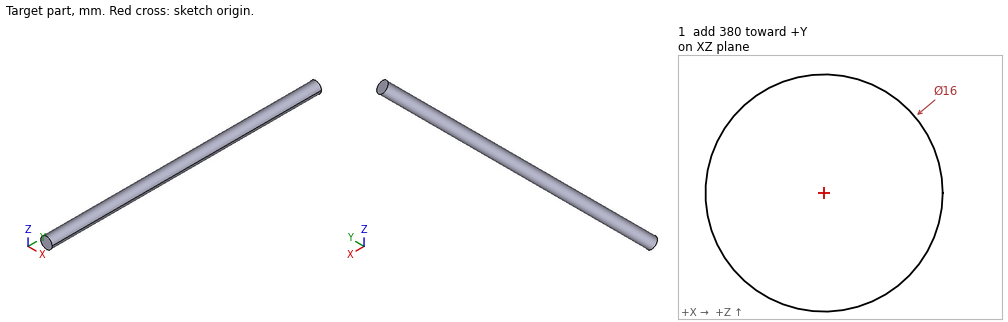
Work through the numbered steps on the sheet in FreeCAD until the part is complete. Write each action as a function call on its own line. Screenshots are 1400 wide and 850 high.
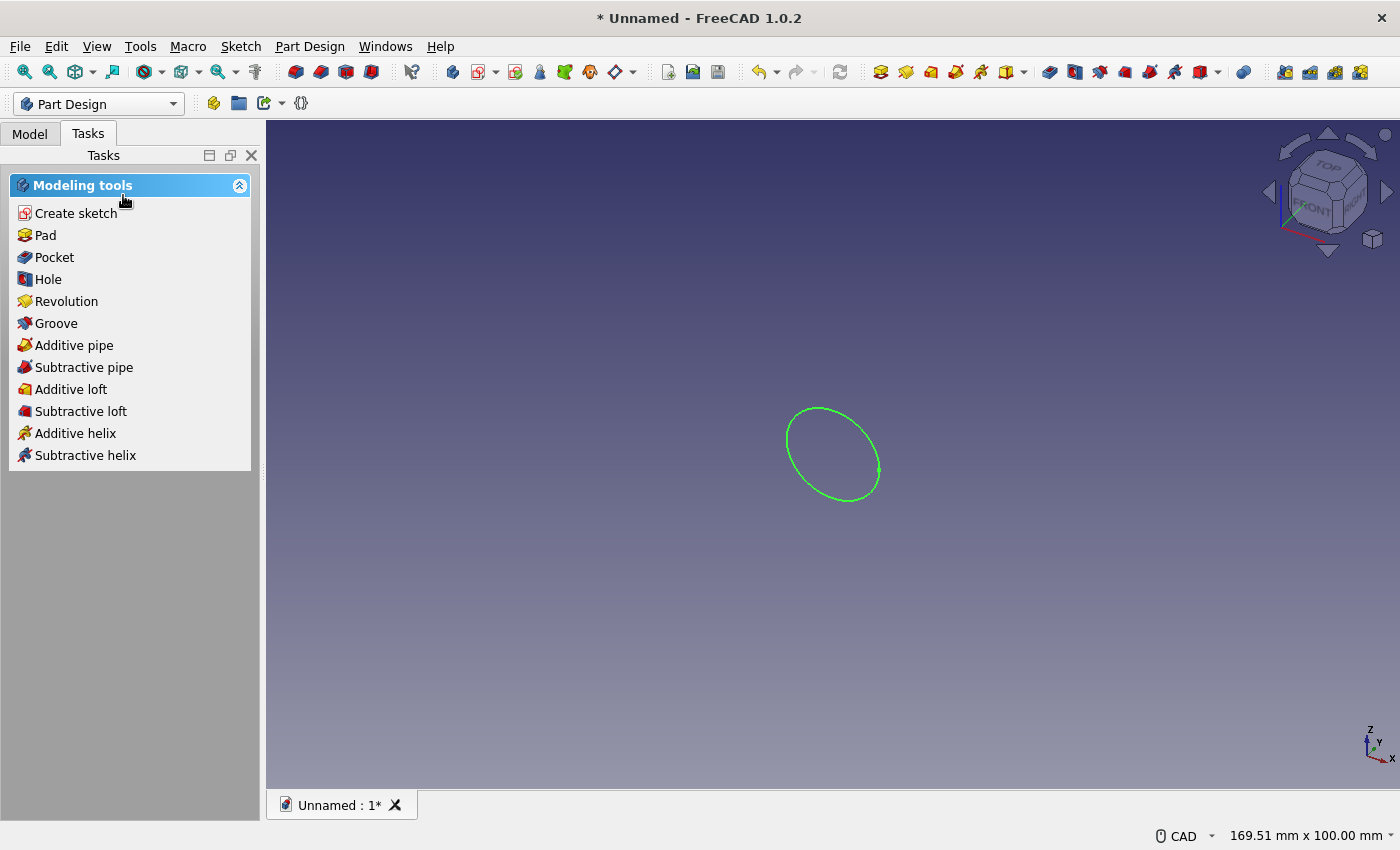
click(881, 72)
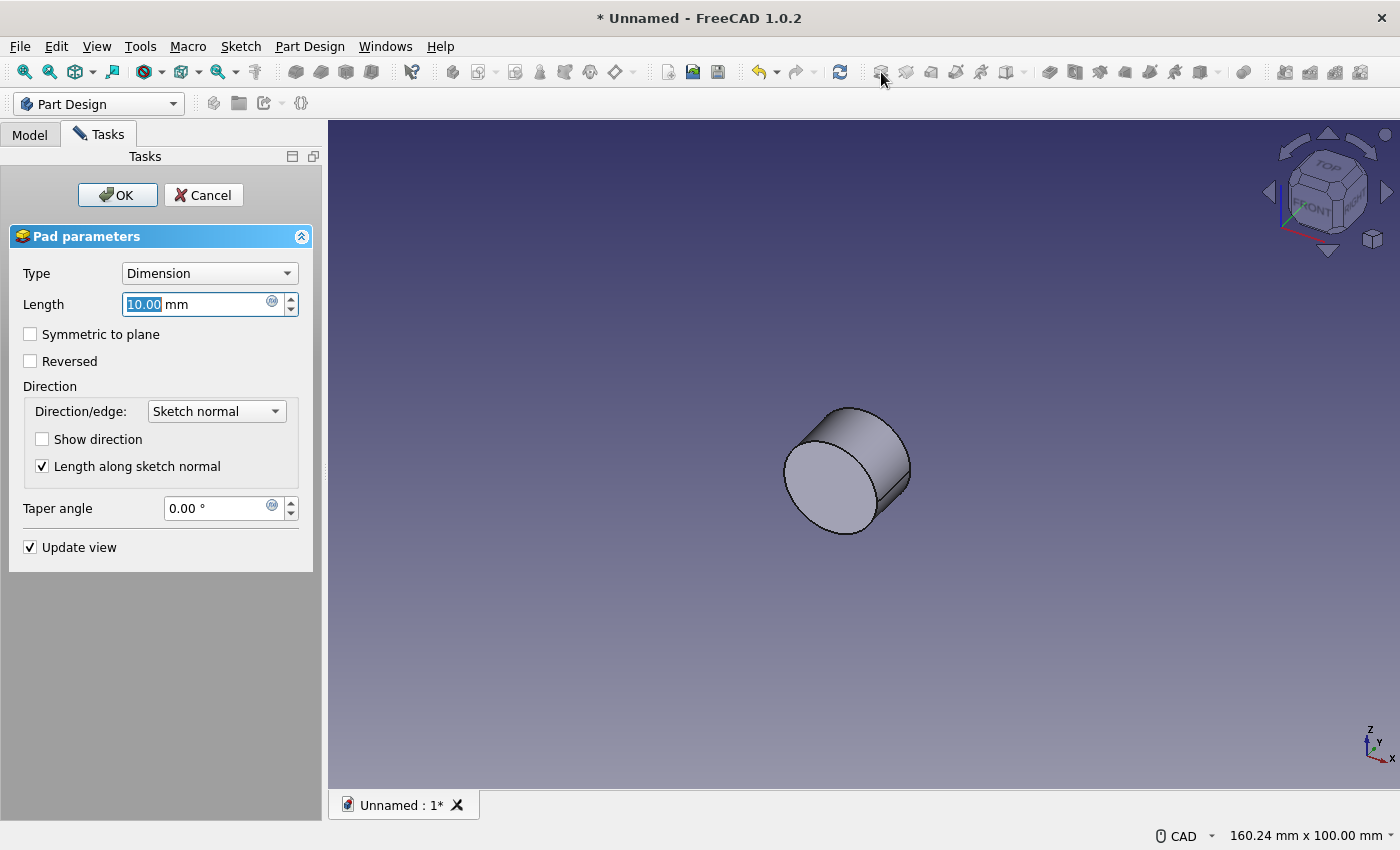
text(380)
key(Tab)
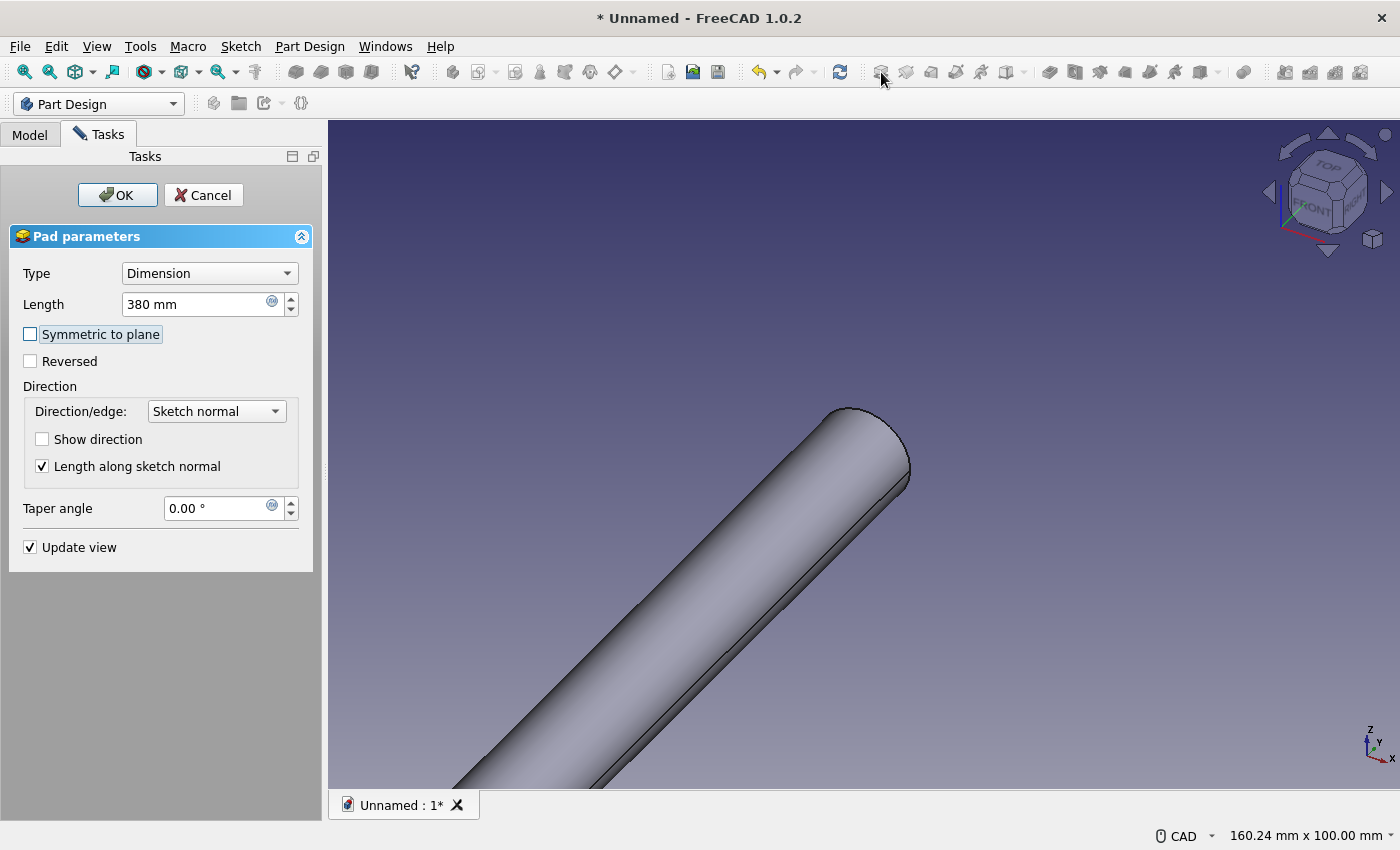
click(31, 361)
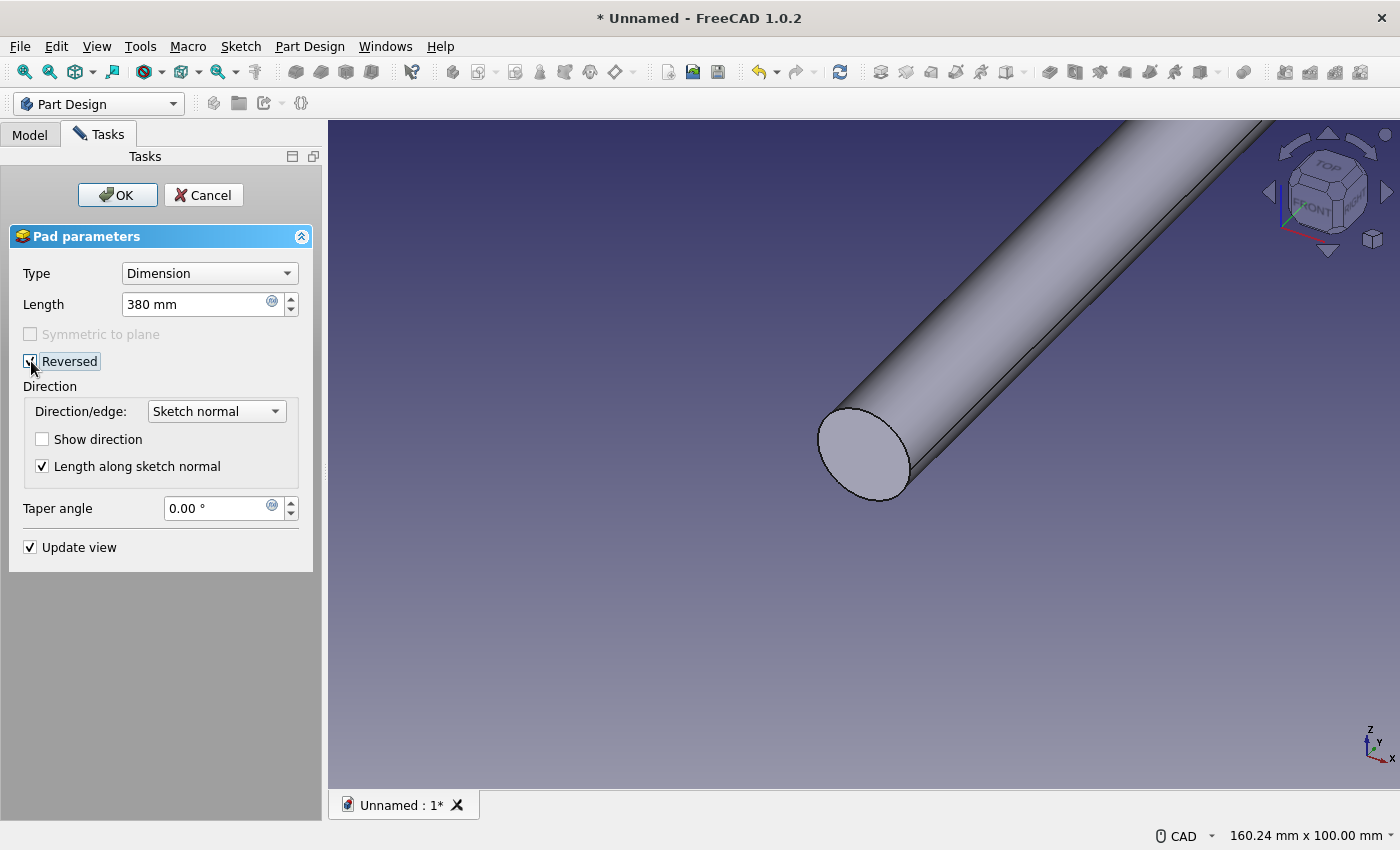
click(118, 195)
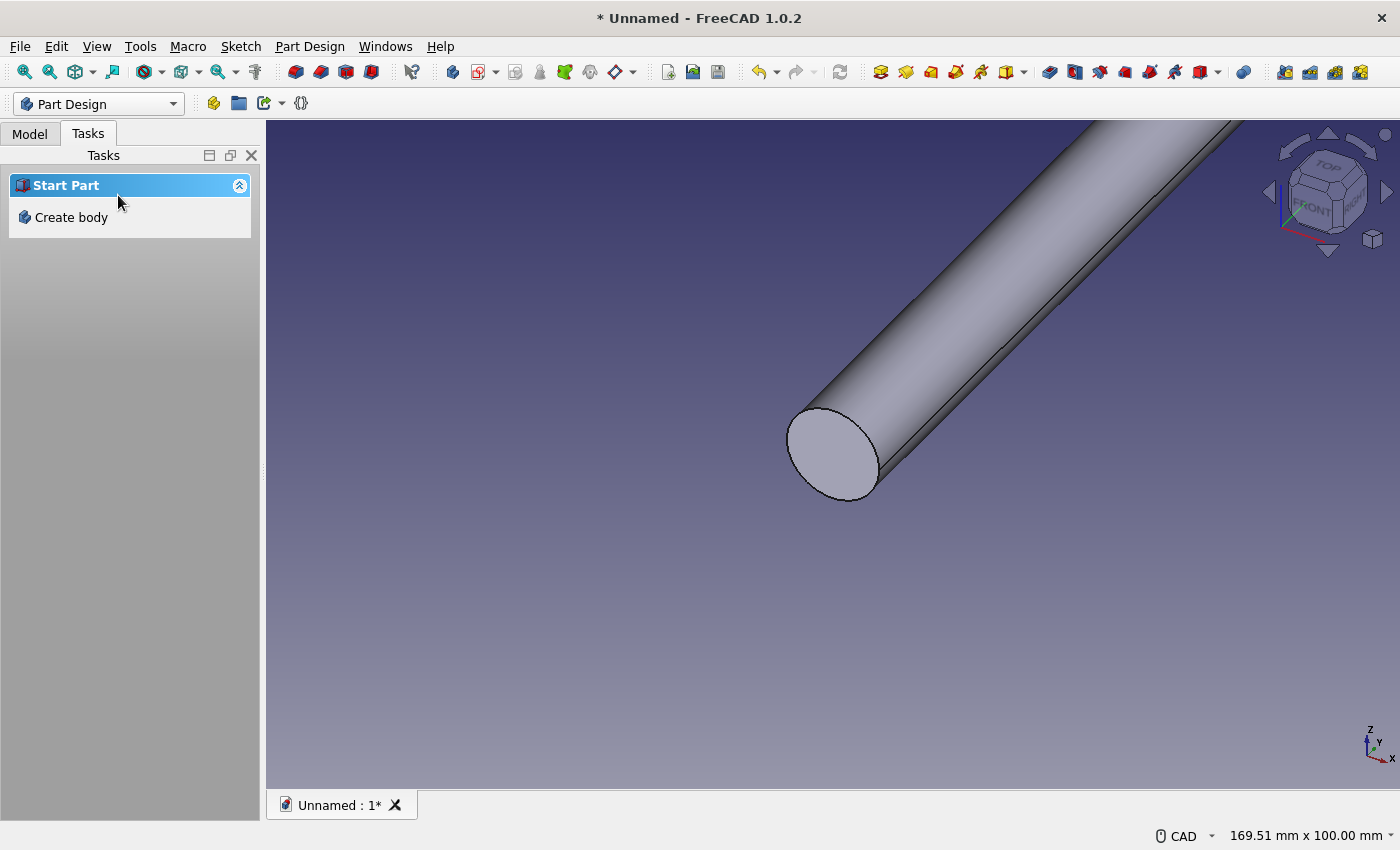
key(0)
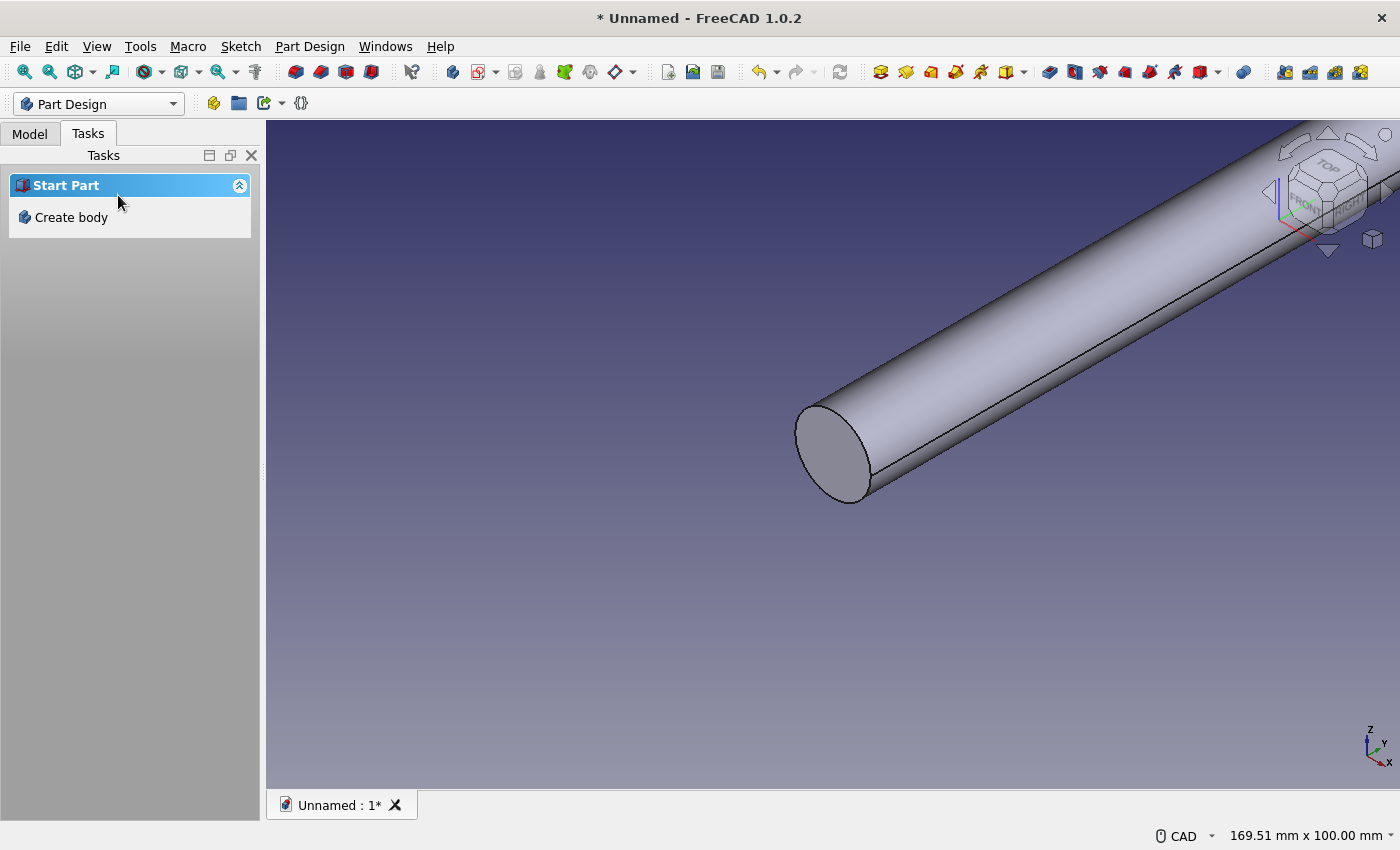
key(v)
key(f)